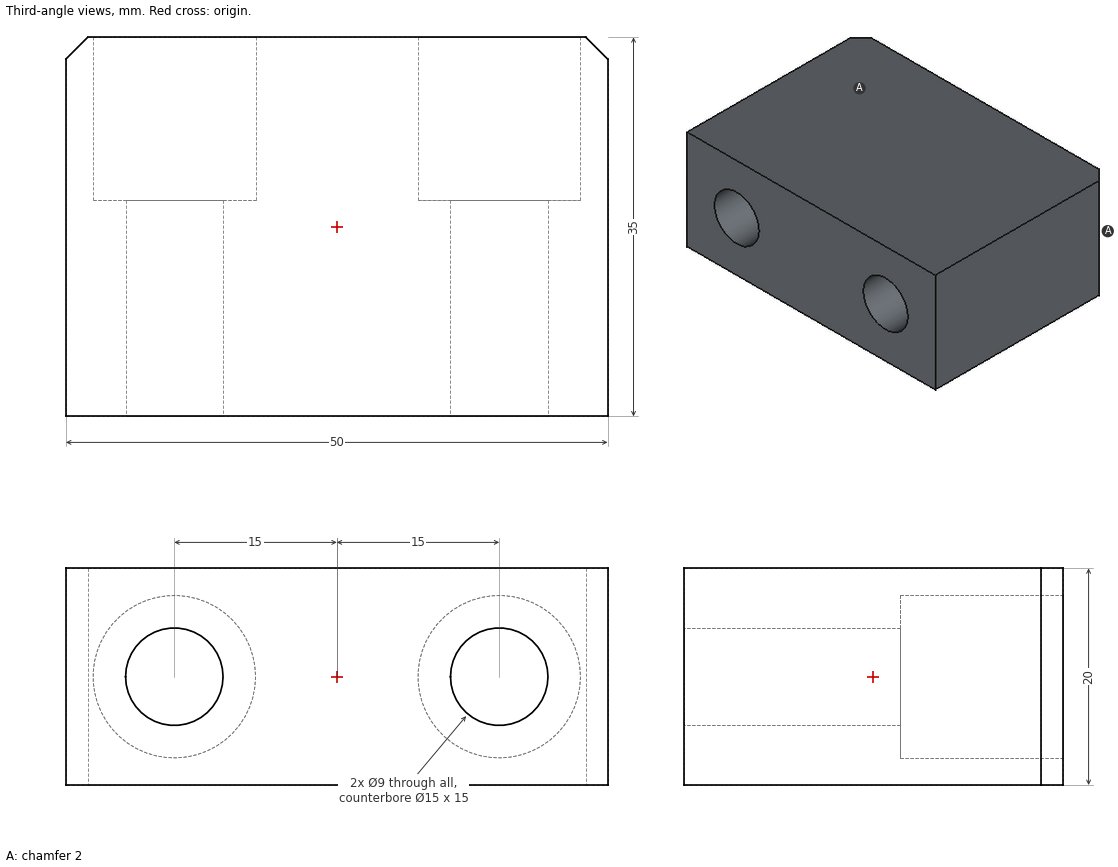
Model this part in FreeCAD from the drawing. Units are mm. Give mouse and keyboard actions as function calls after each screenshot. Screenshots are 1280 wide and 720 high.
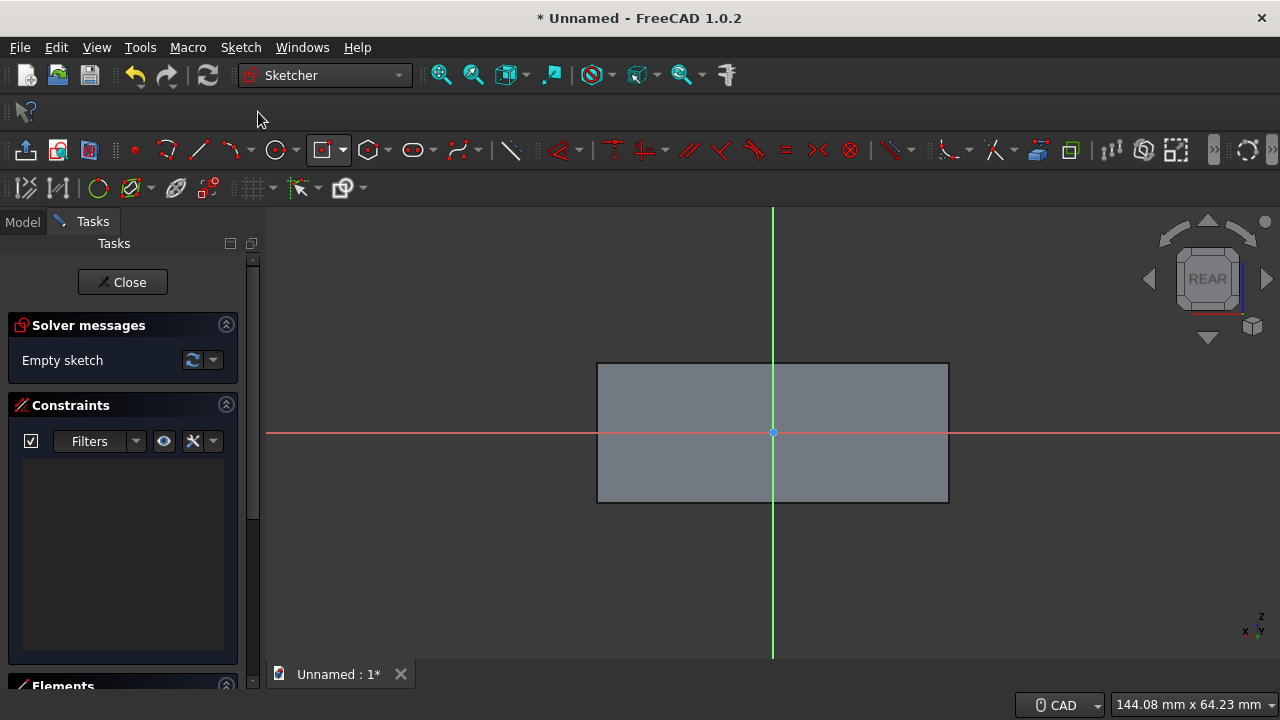
scroll(829, 433, up, 4)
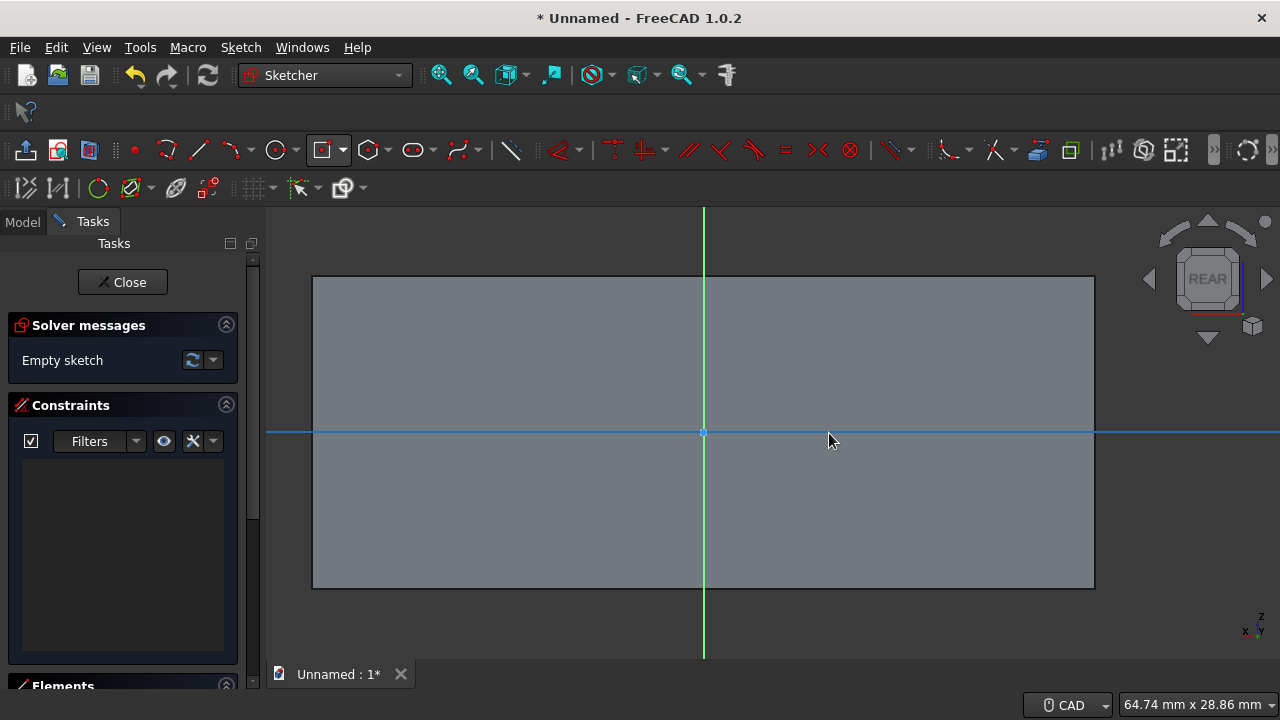
click(276, 150)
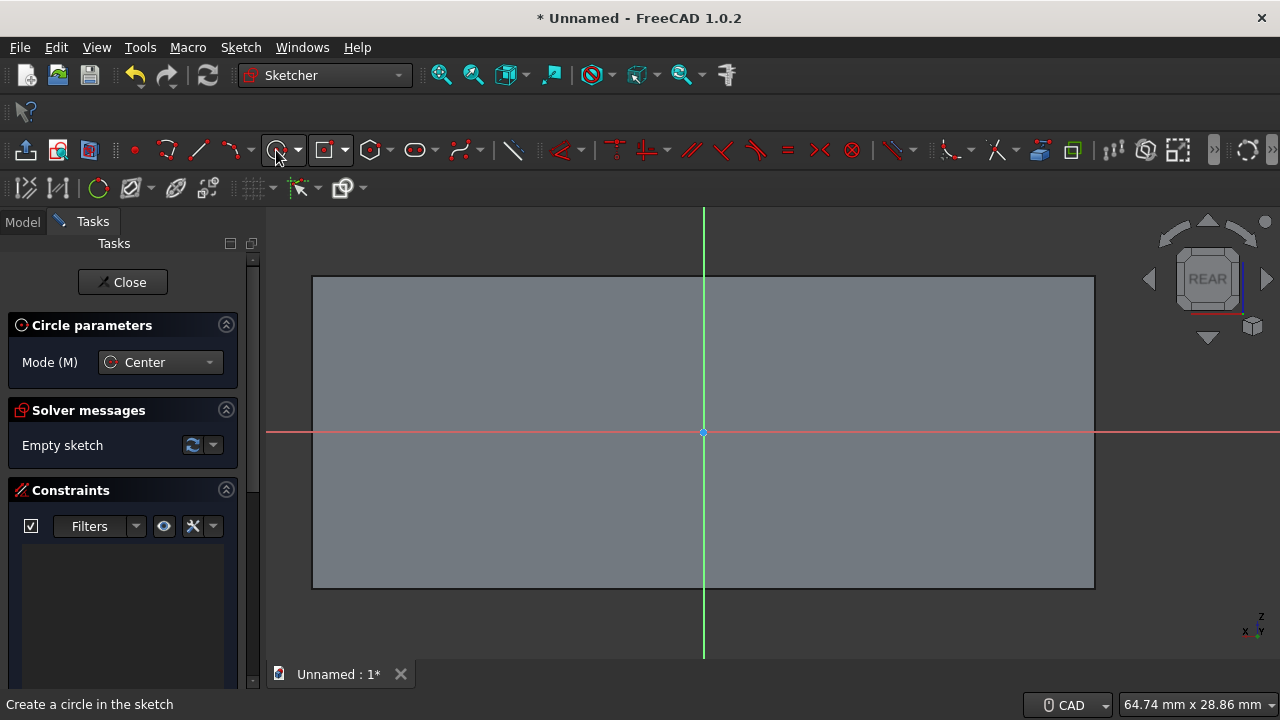
click(469, 432)
click(519, 383)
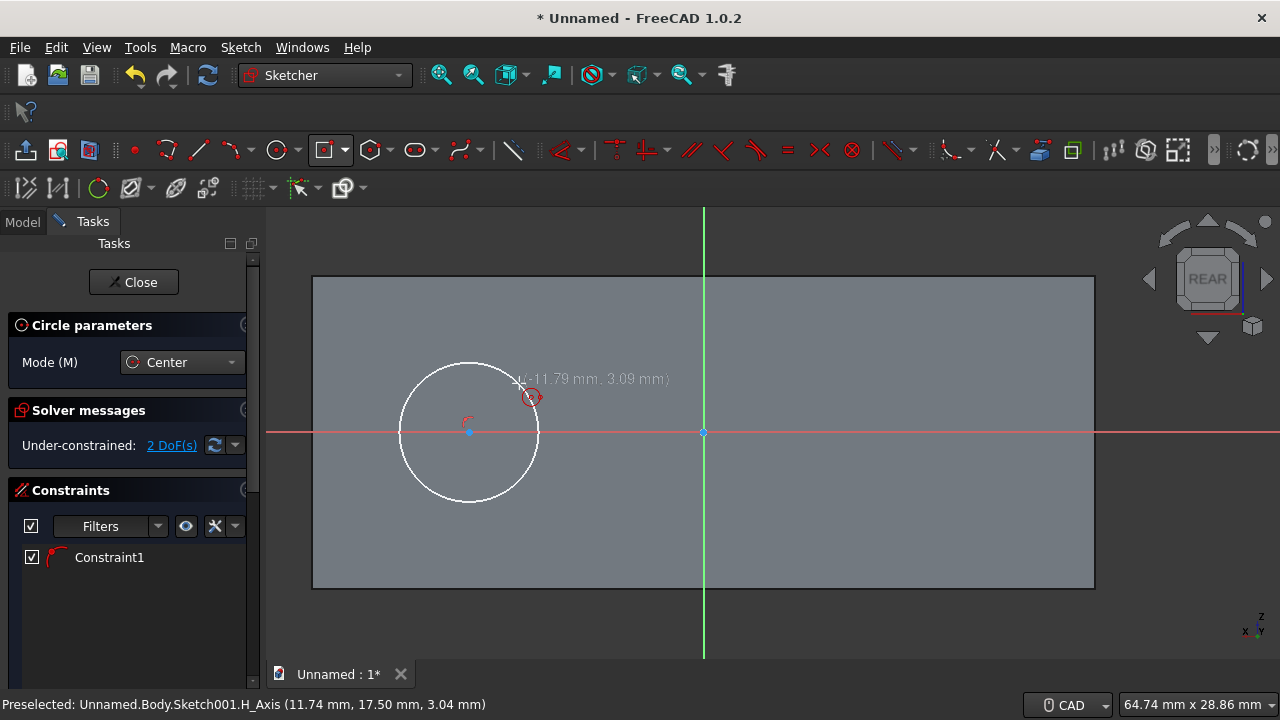
click(939, 432)
click(988, 383)
key(Escape)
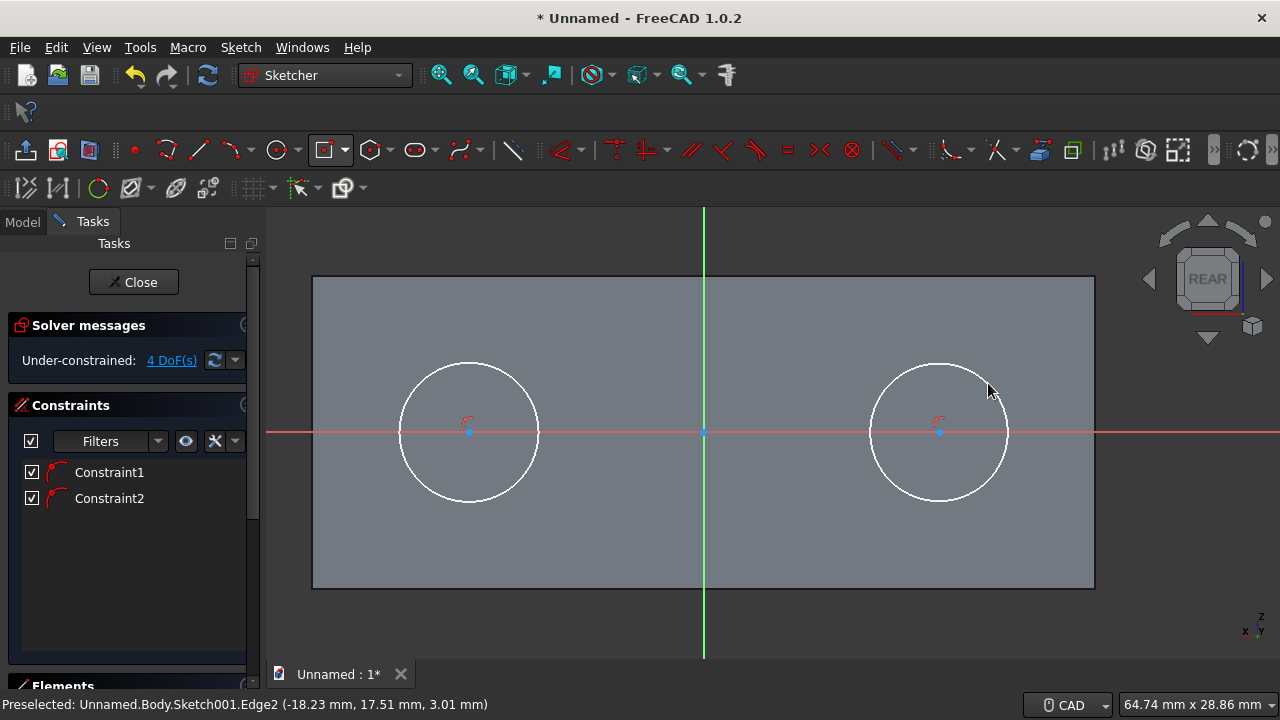
click(518, 383)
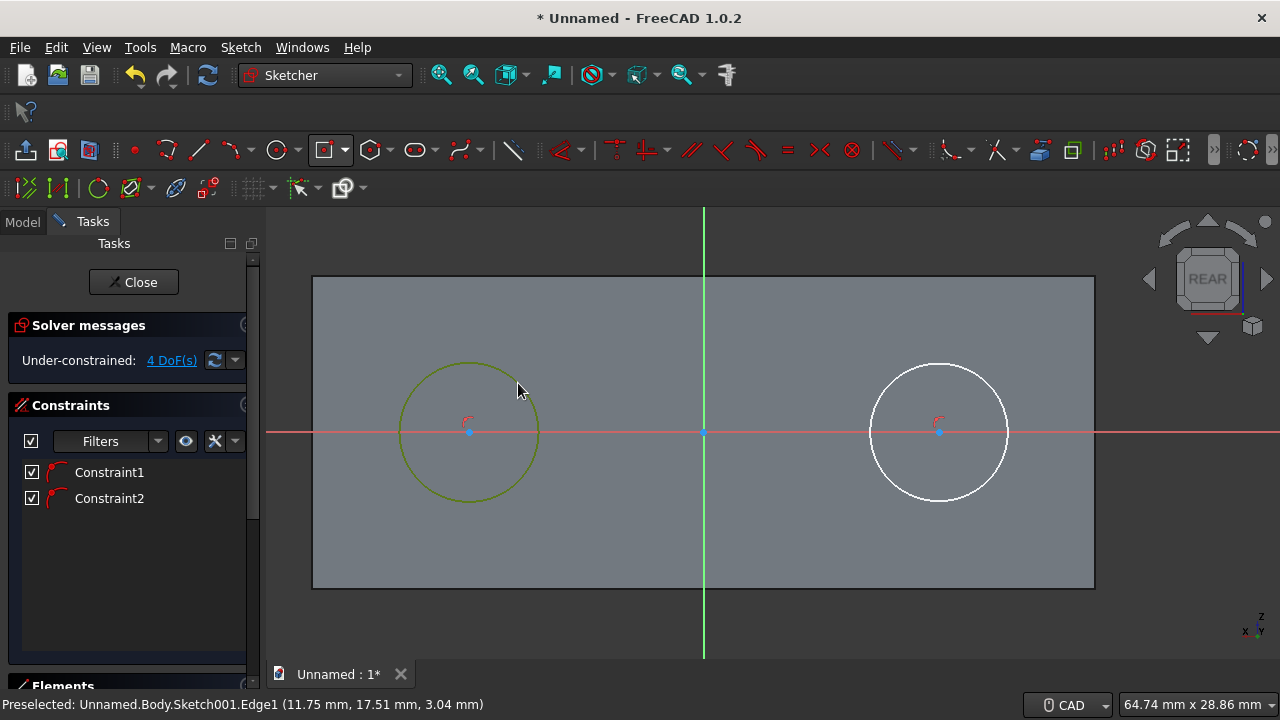
click(988, 384)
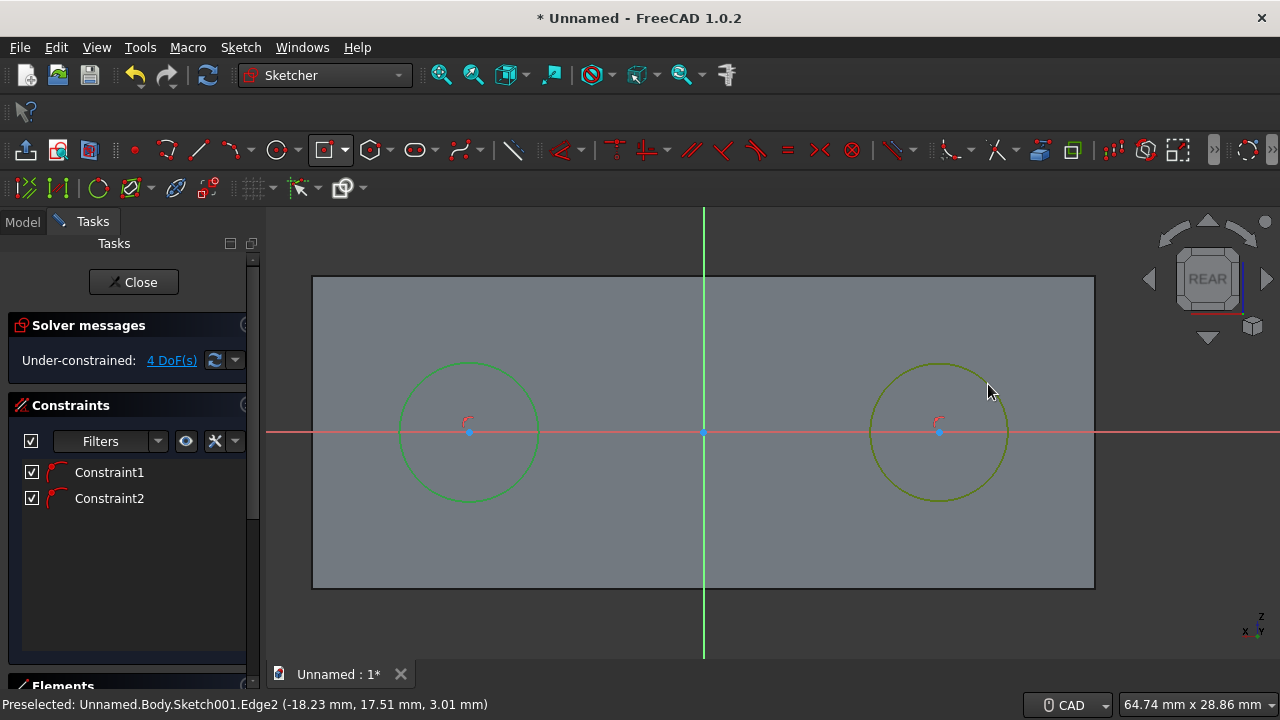
click(788, 150)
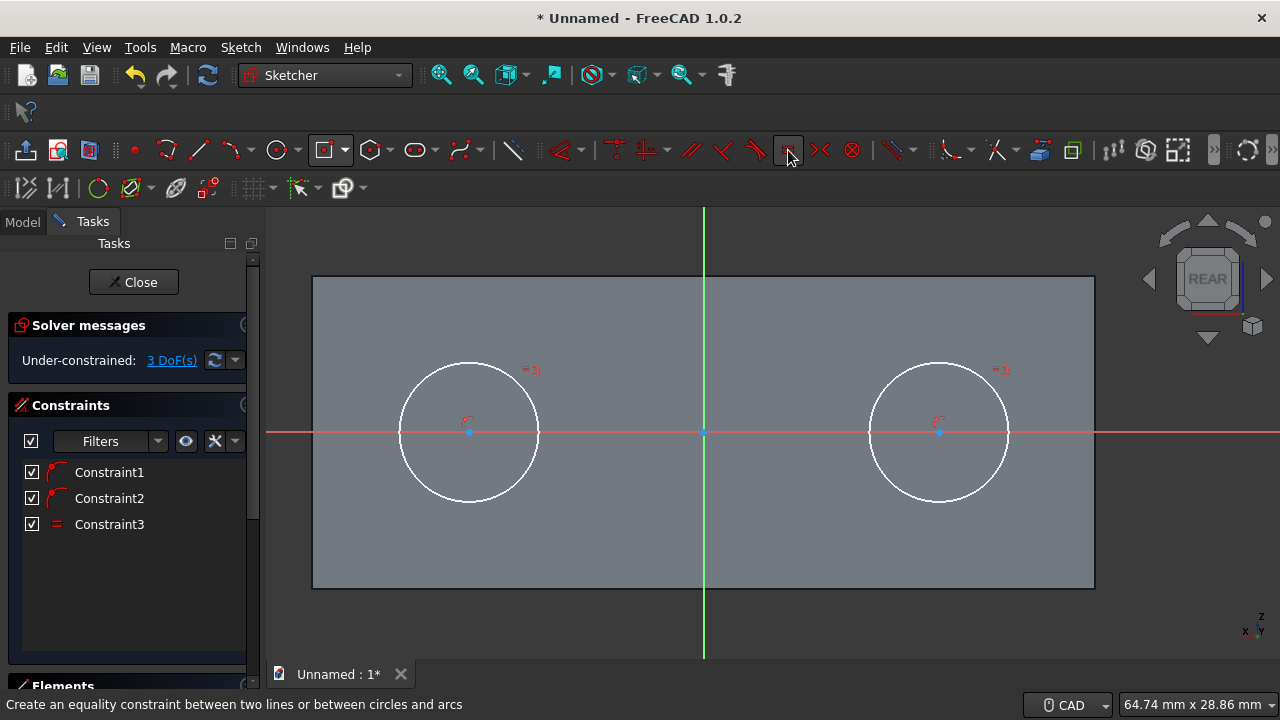
click(560, 150)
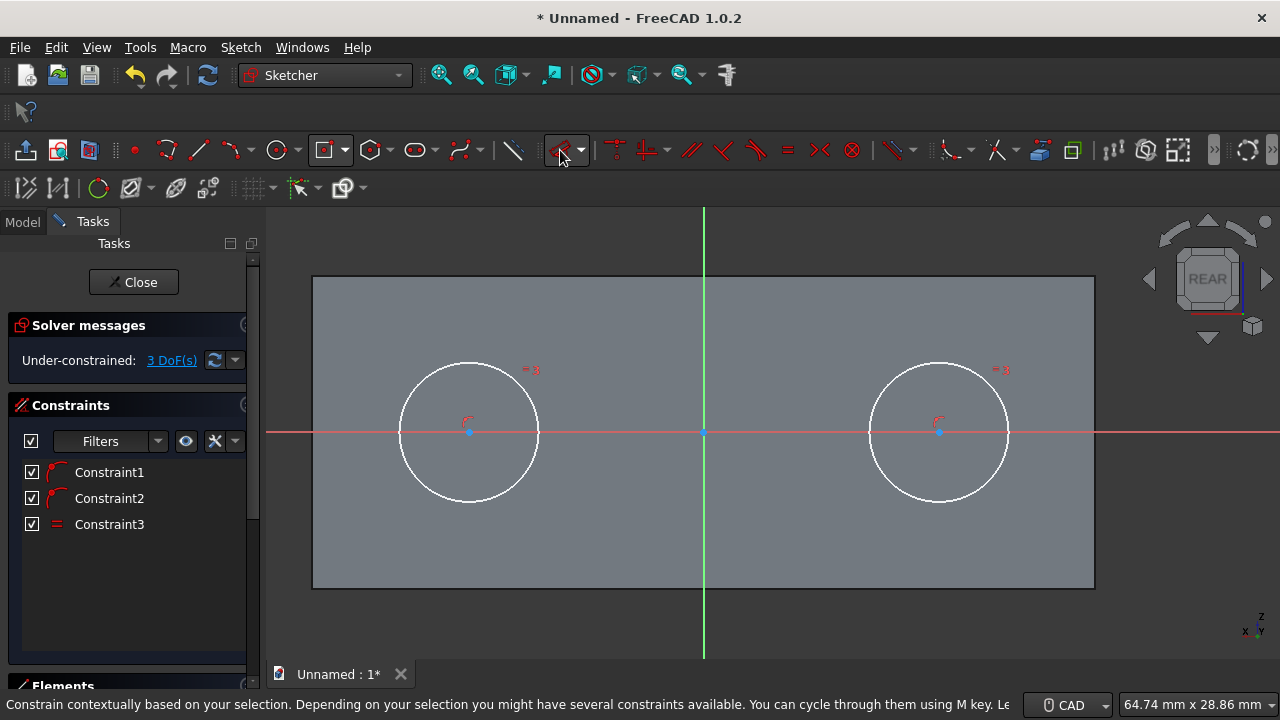
click(518, 383)
click(541, 360)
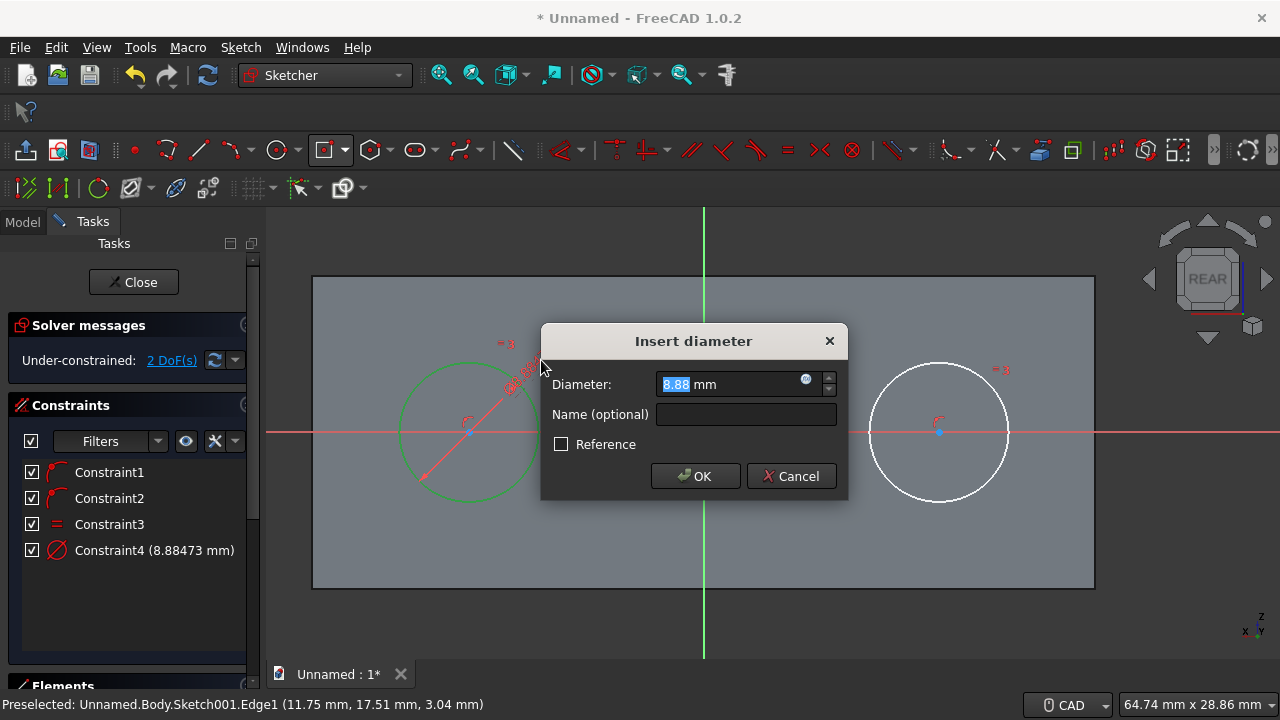
text(9)
key(Return)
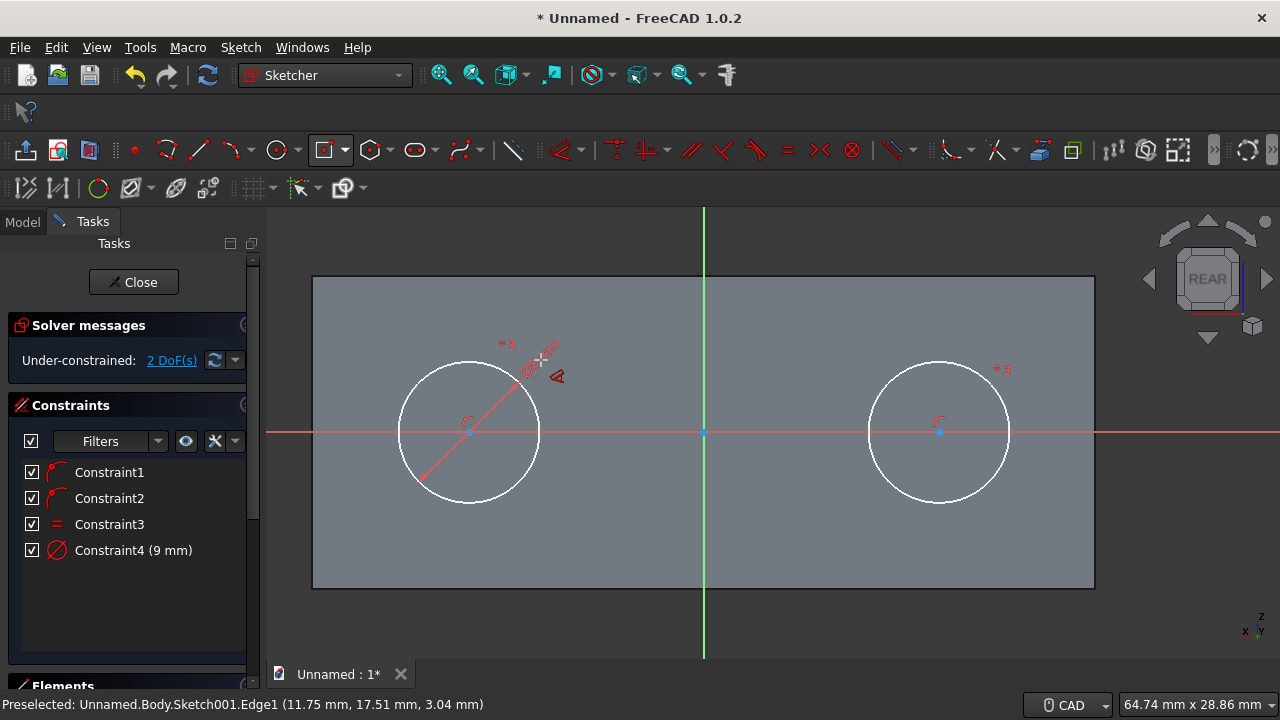
click(469, 432)
click(586, 466)